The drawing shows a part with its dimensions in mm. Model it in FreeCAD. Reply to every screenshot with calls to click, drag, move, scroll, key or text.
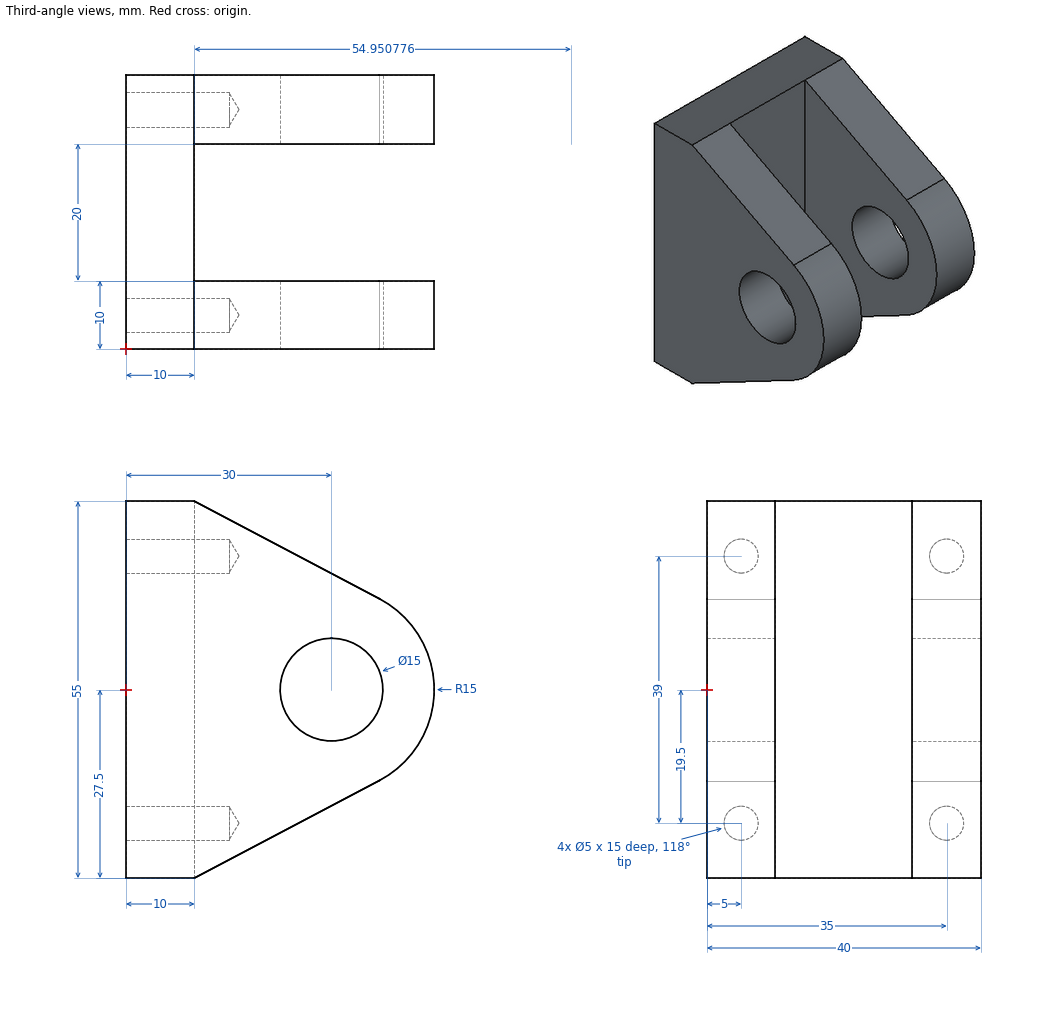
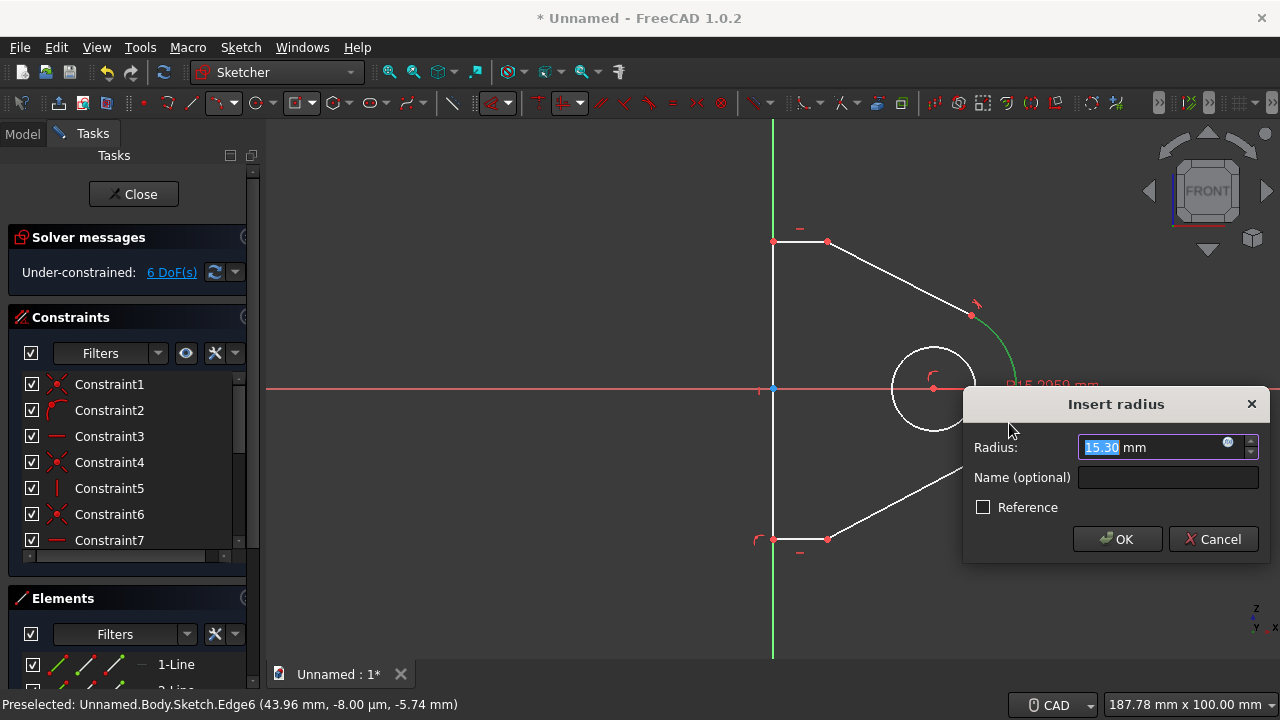
text(15)
key(Return)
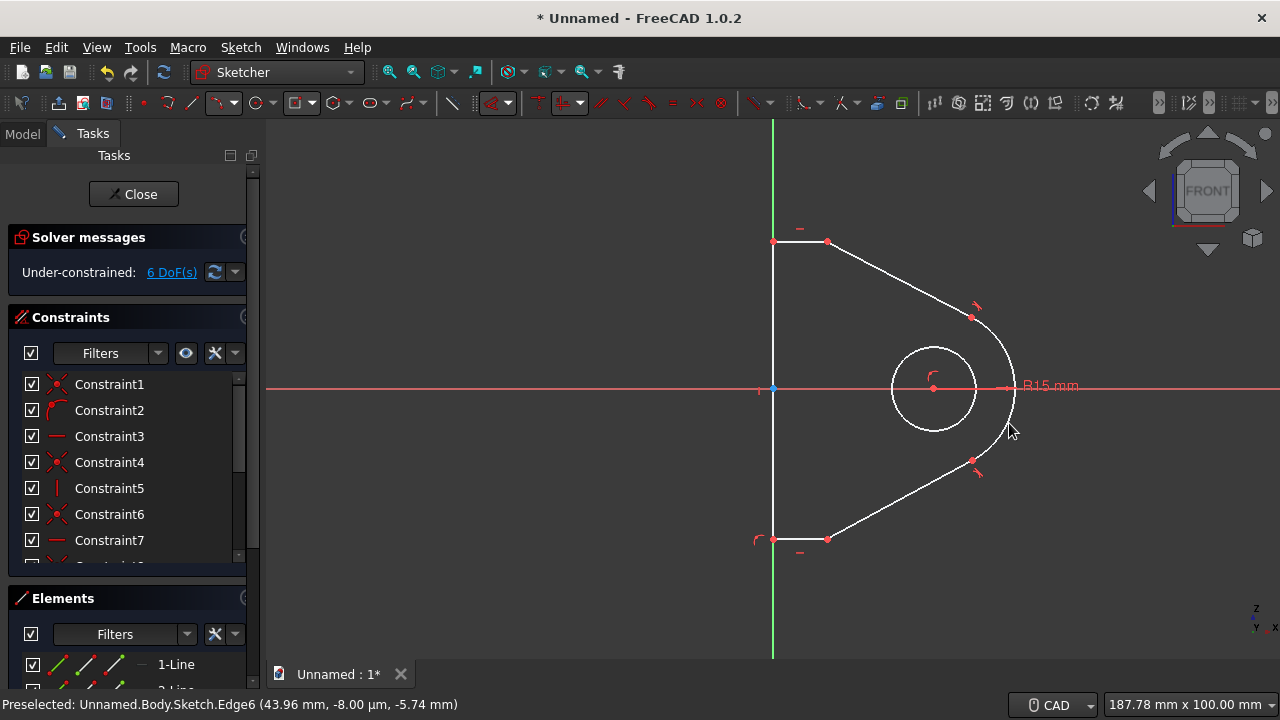
click(963, 359)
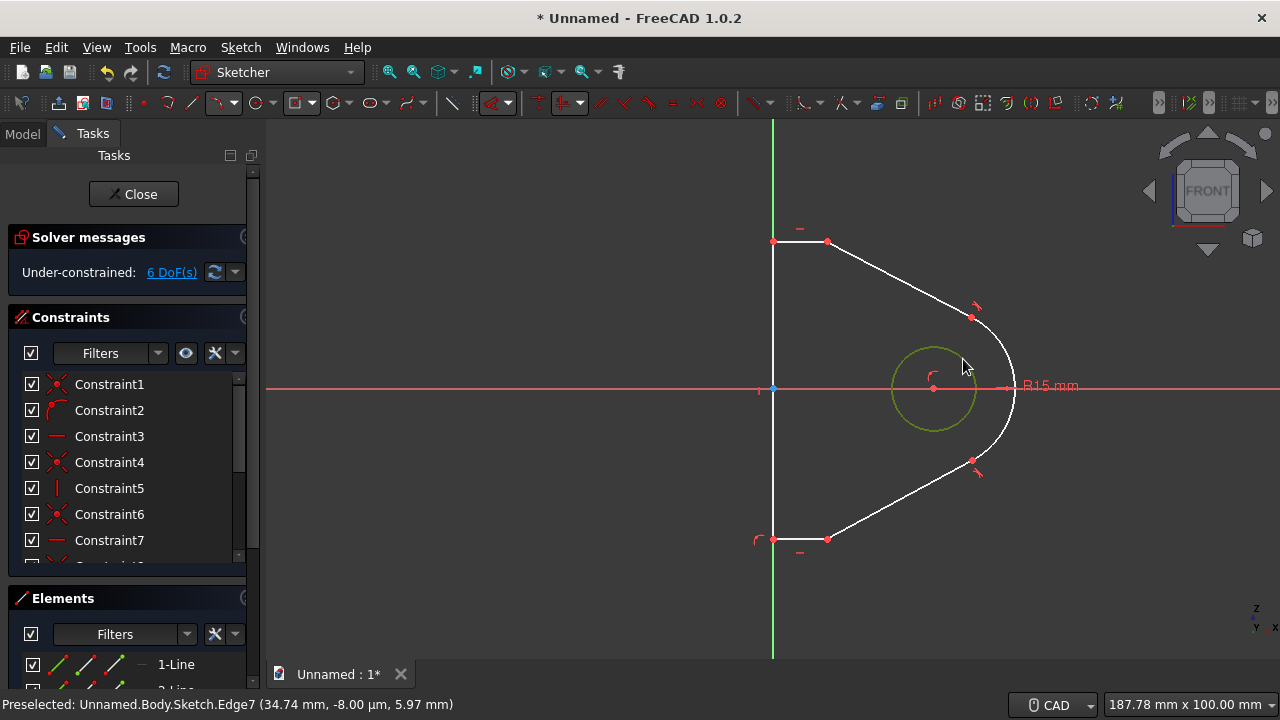
key(k)
key(o)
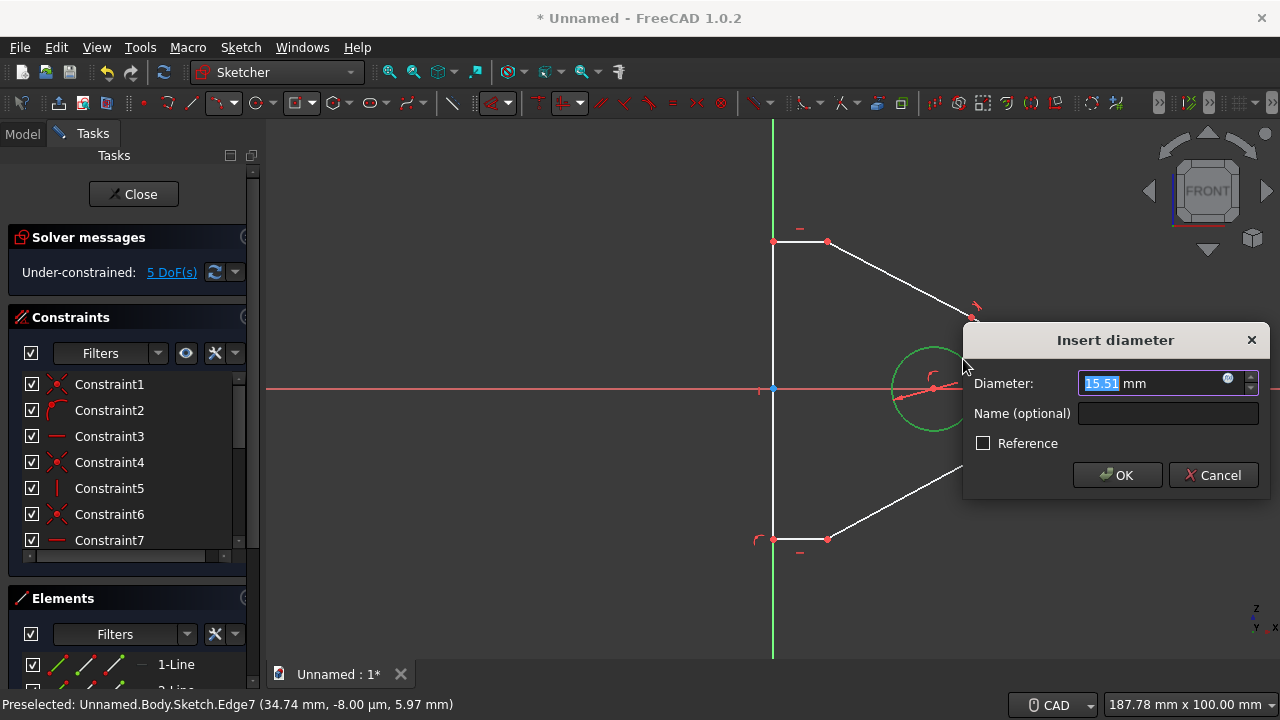
text(15)
key(Return)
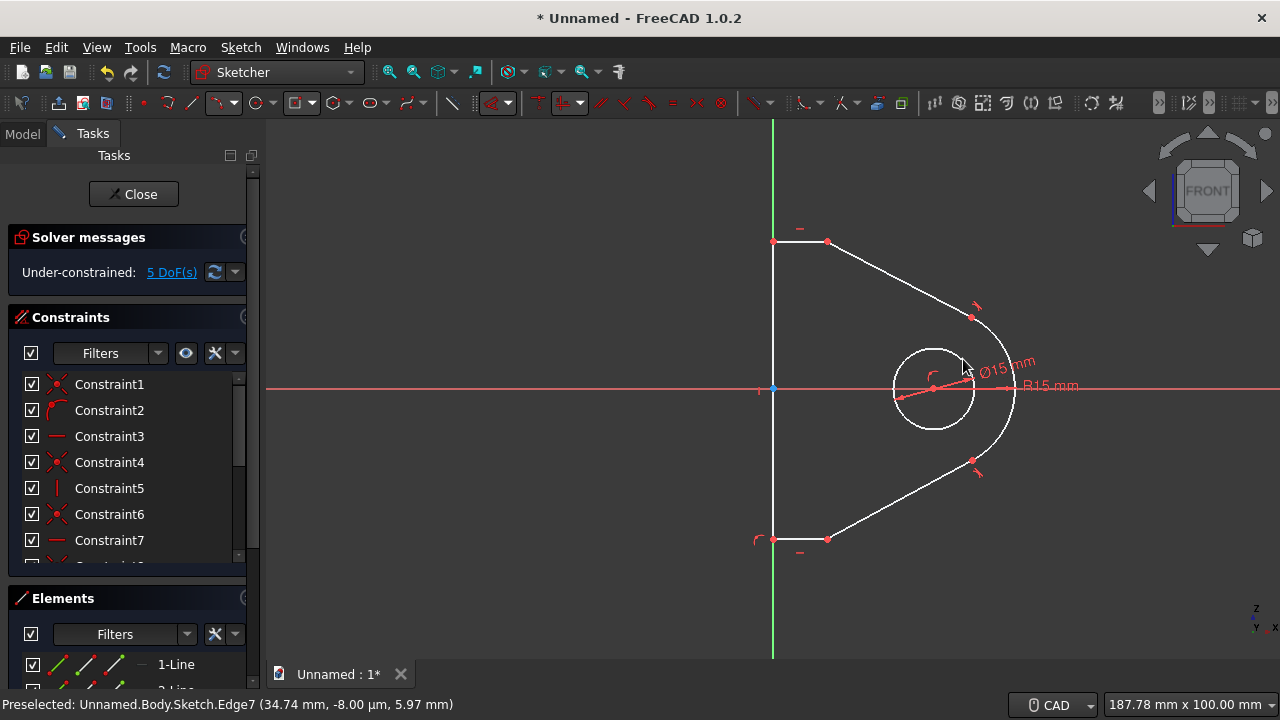
click(811, 539)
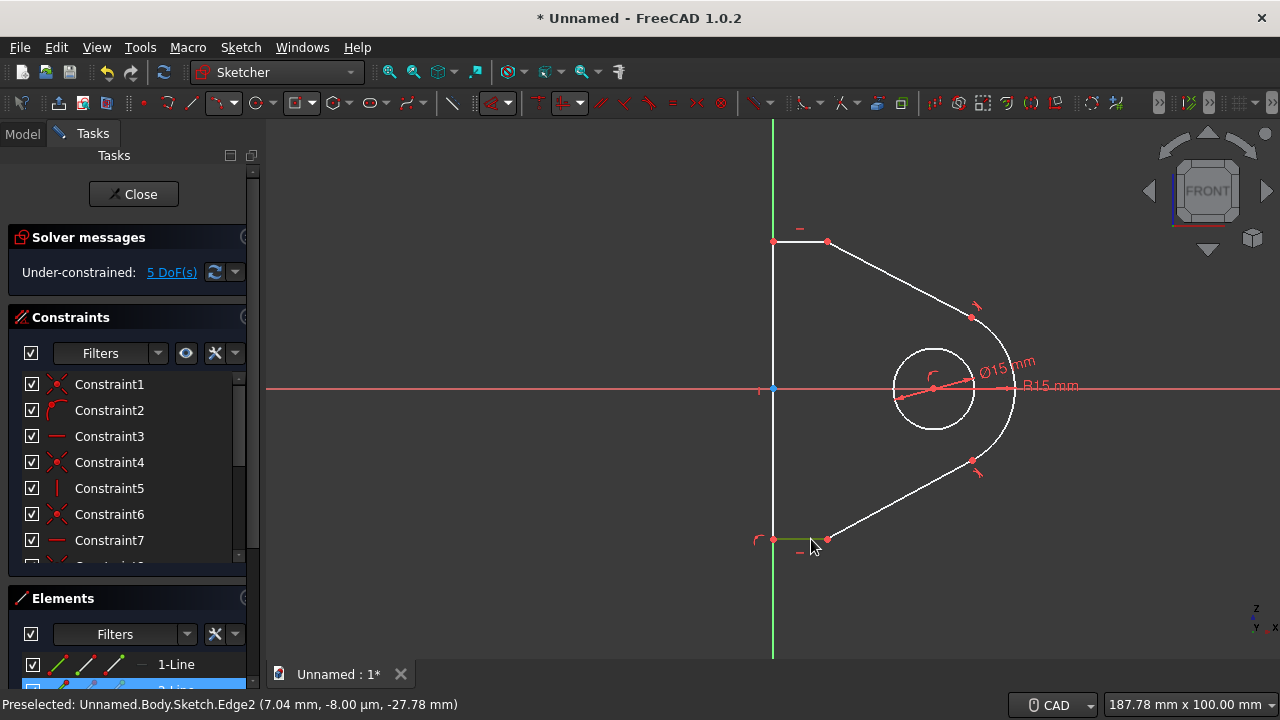
click(510, 104)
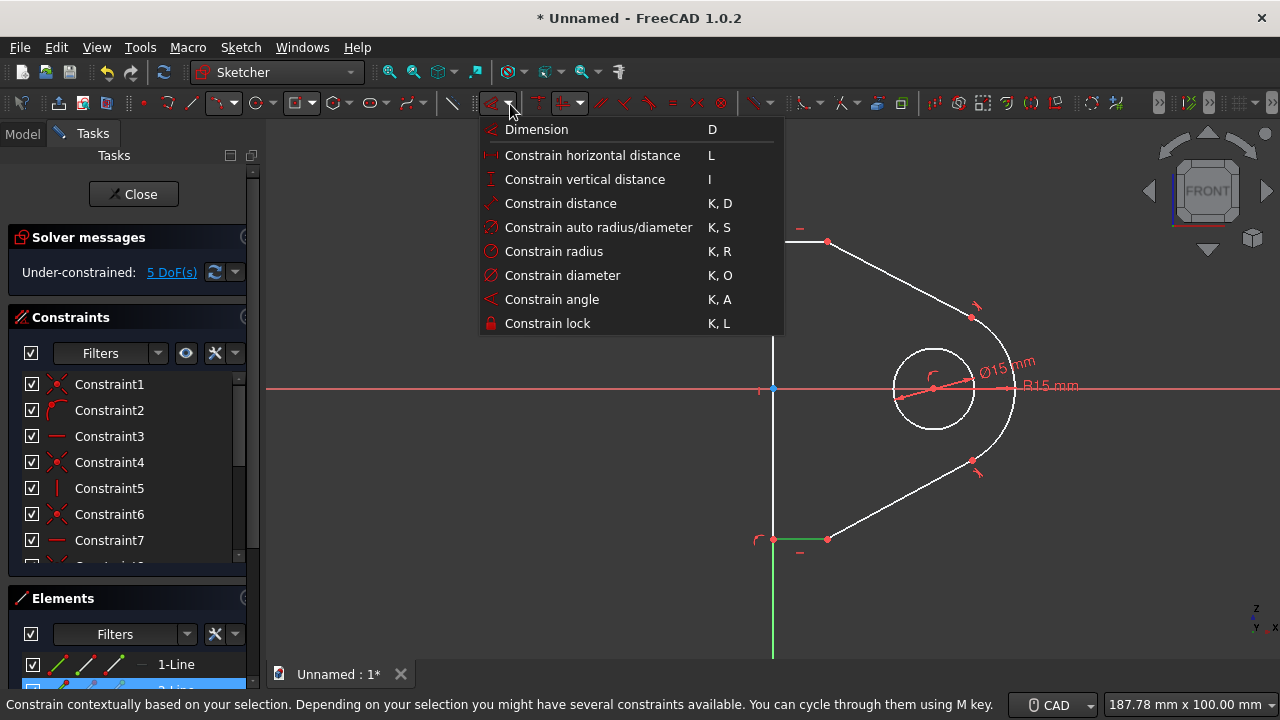
click(632, 155)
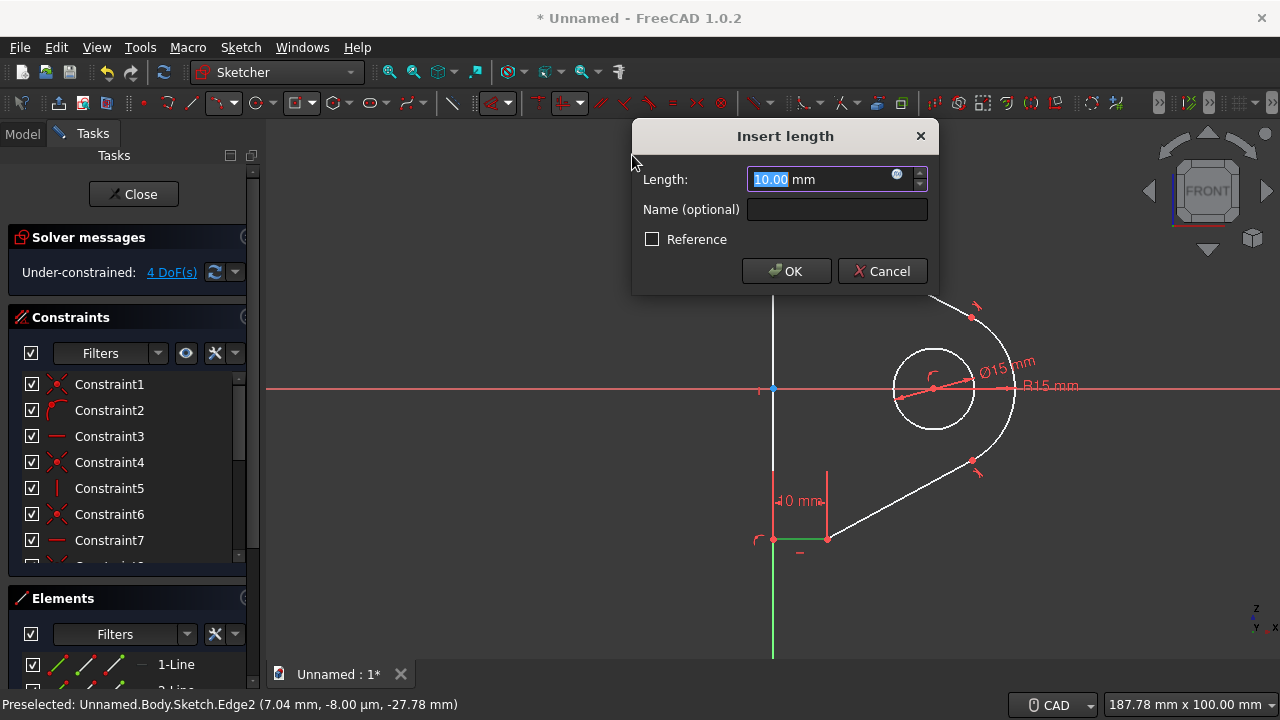
text(10)
key(Return)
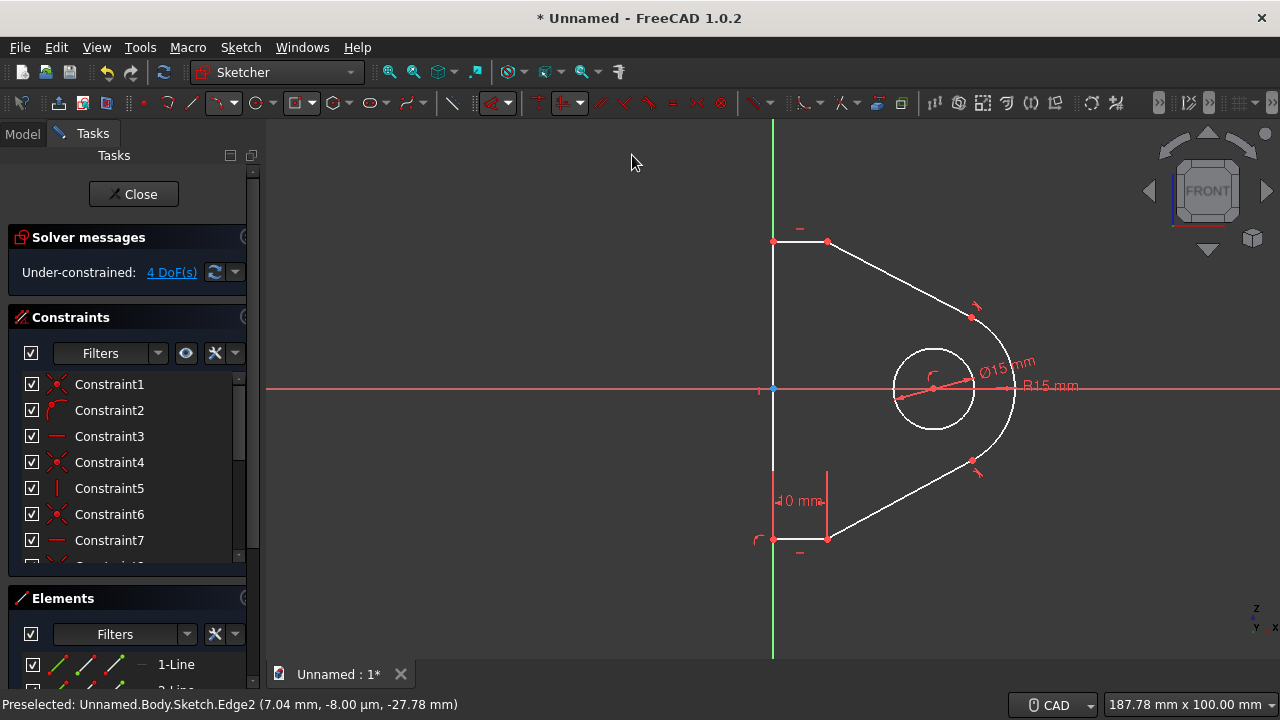
click(773, 450)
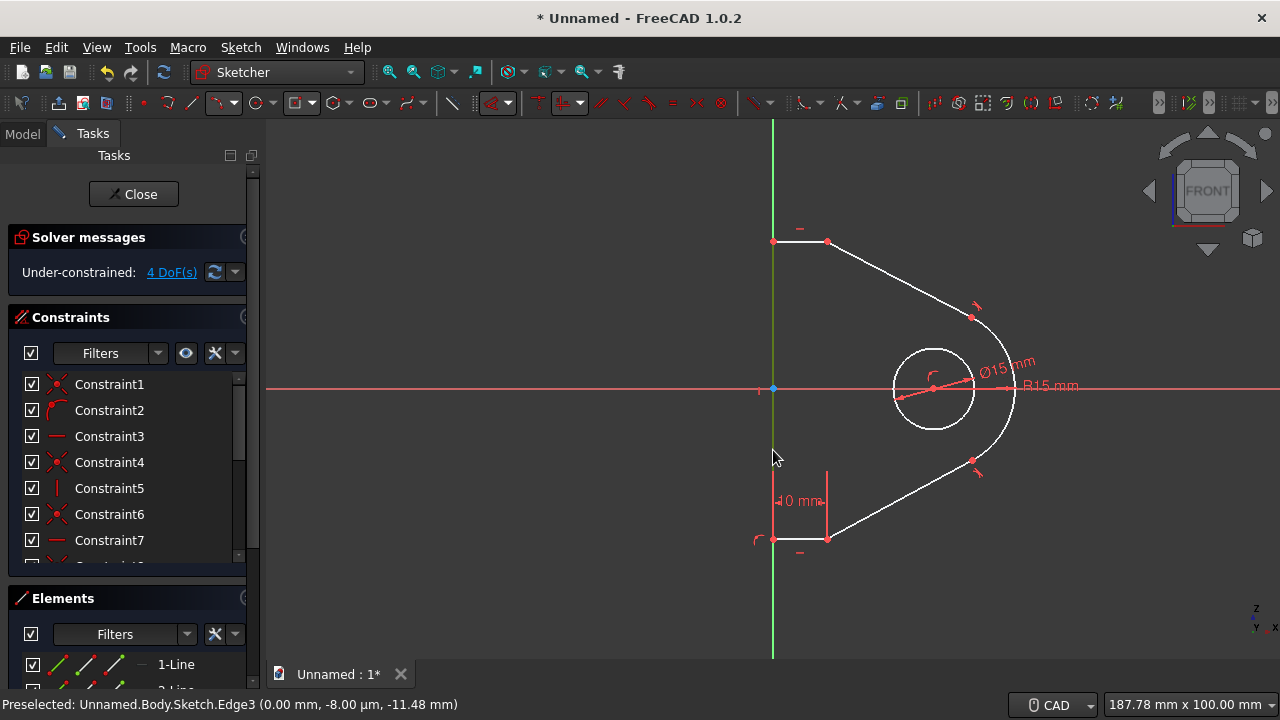
key(i)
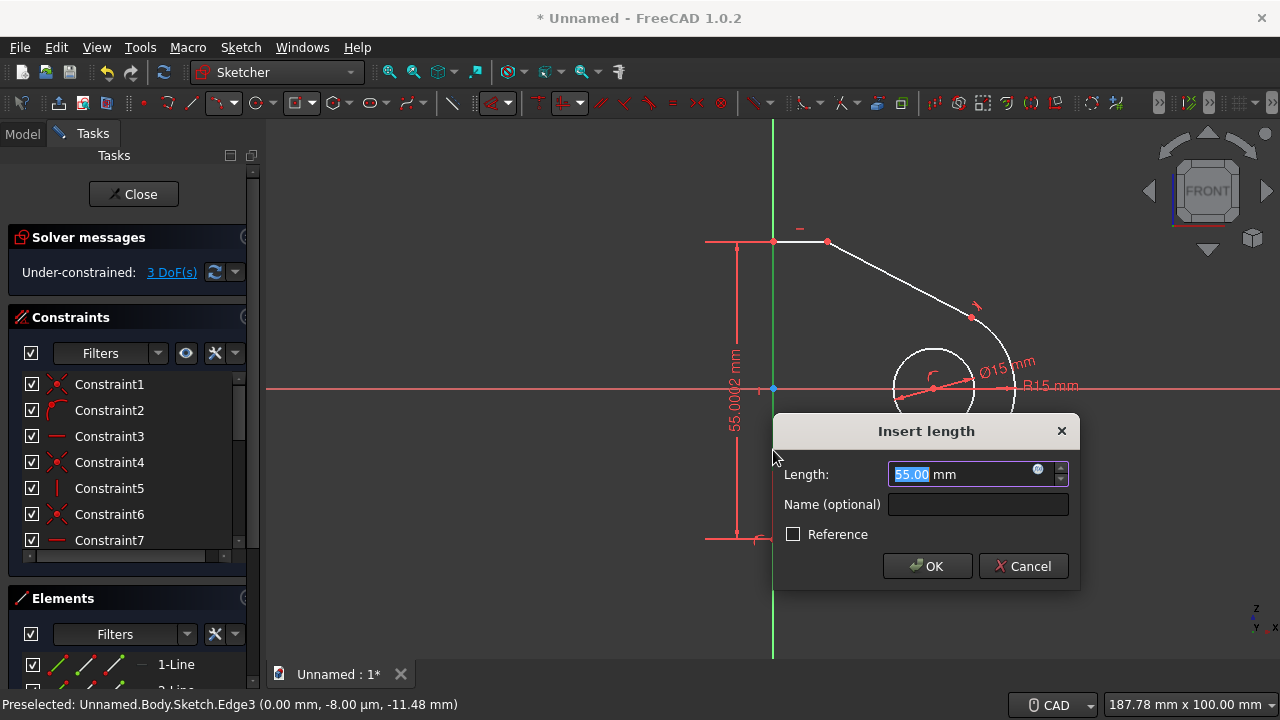
text(55)
key(Return)